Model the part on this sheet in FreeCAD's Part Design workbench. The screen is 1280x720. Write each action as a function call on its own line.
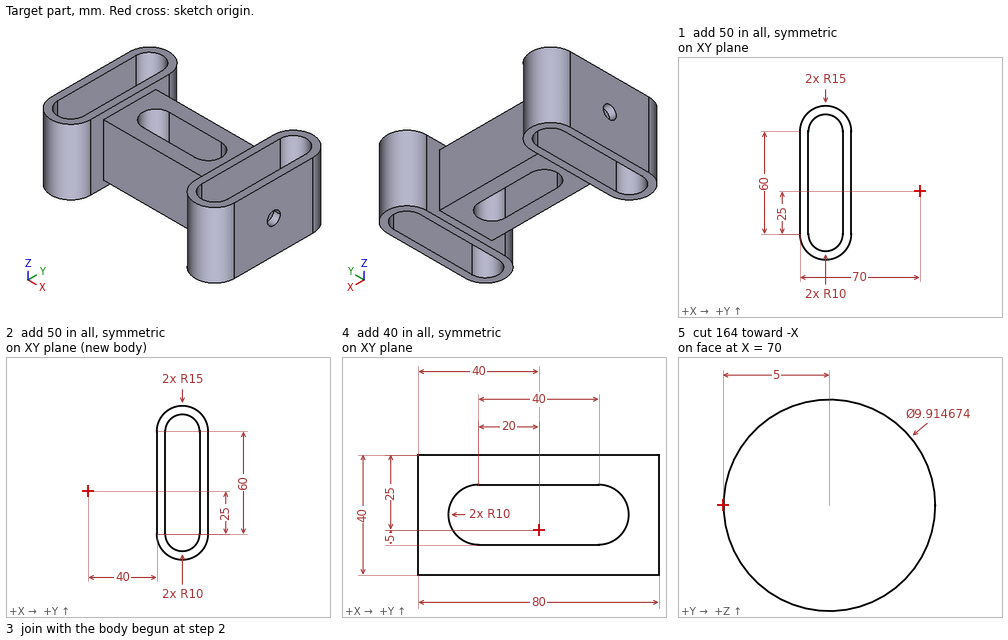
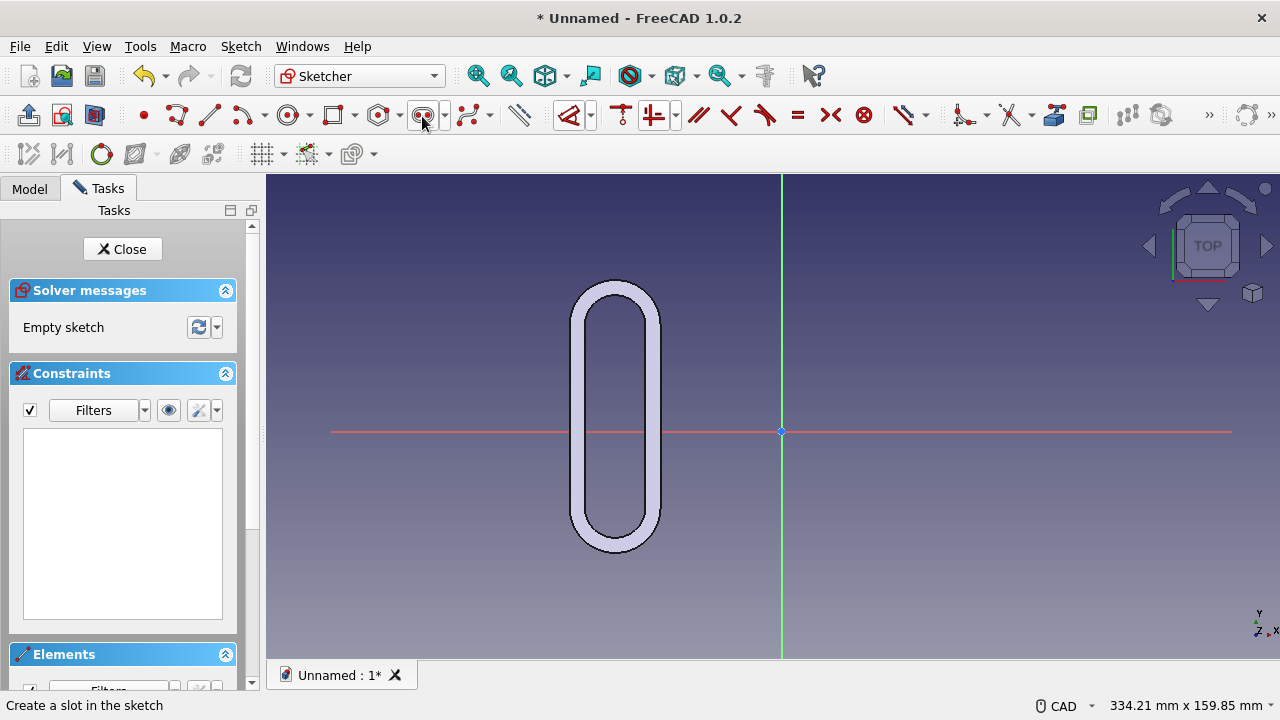
click(949, 508)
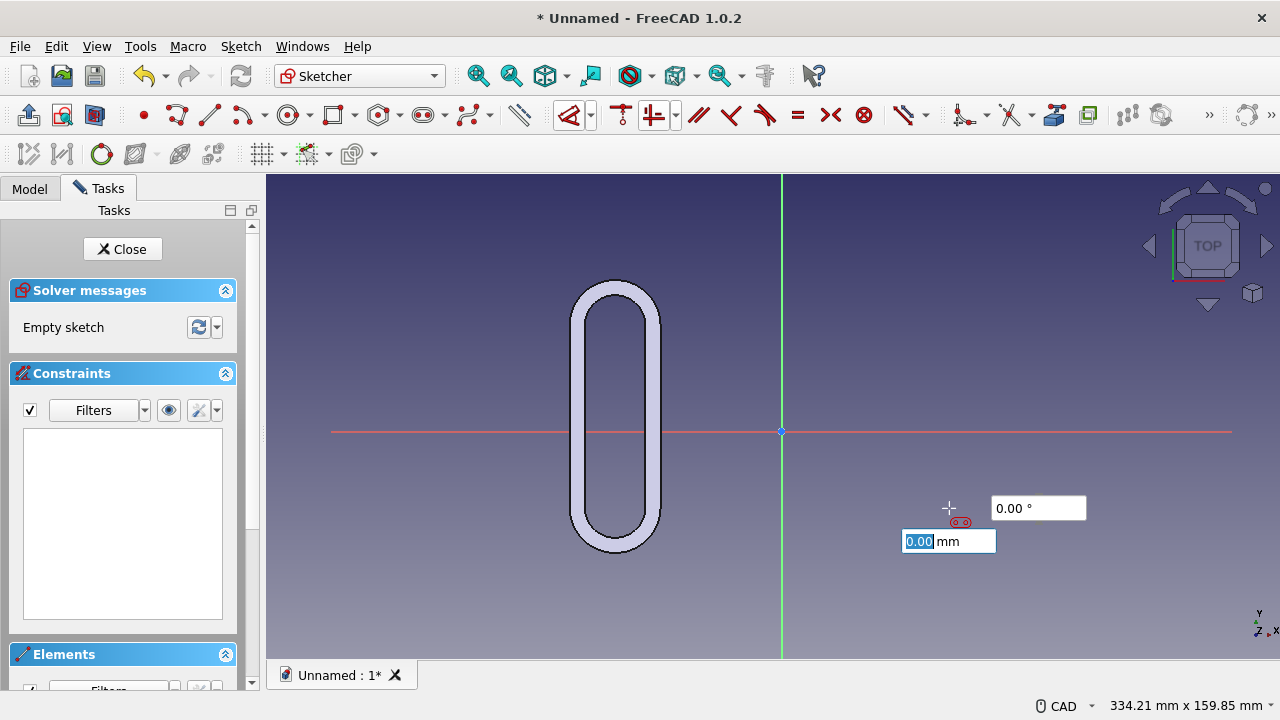
click(949, 325)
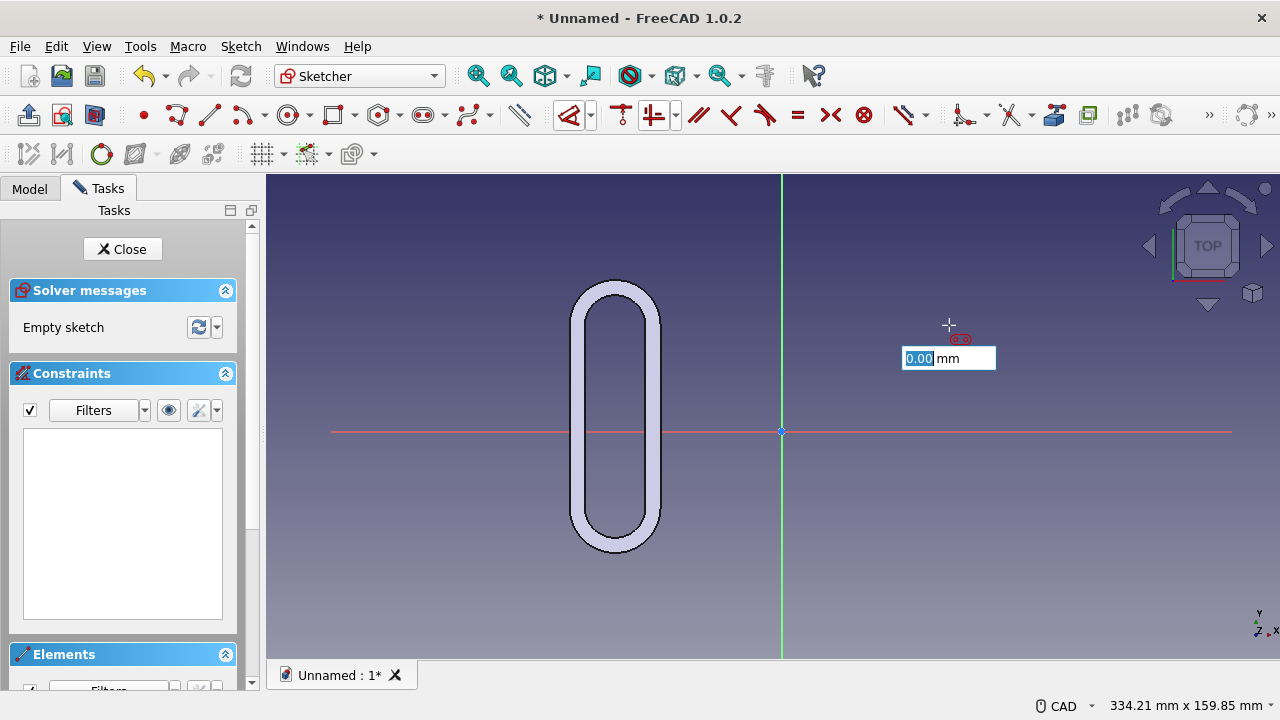
click(994, 416)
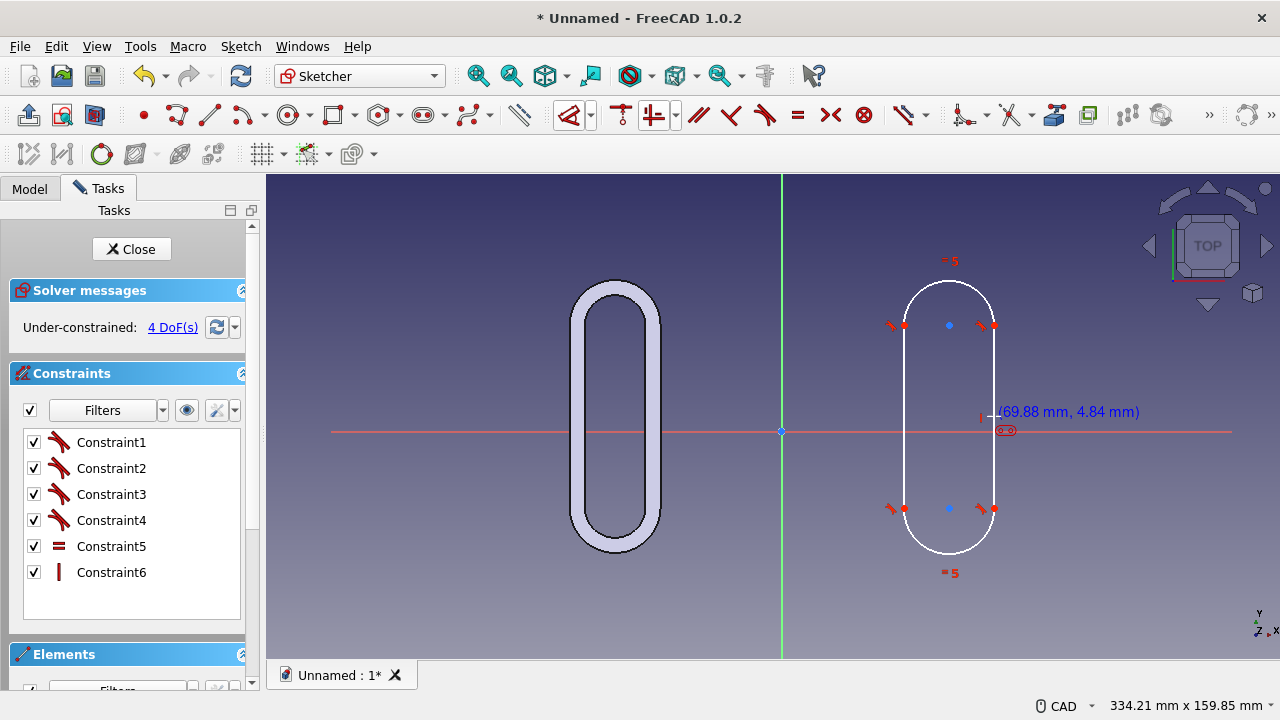
click(949, 509)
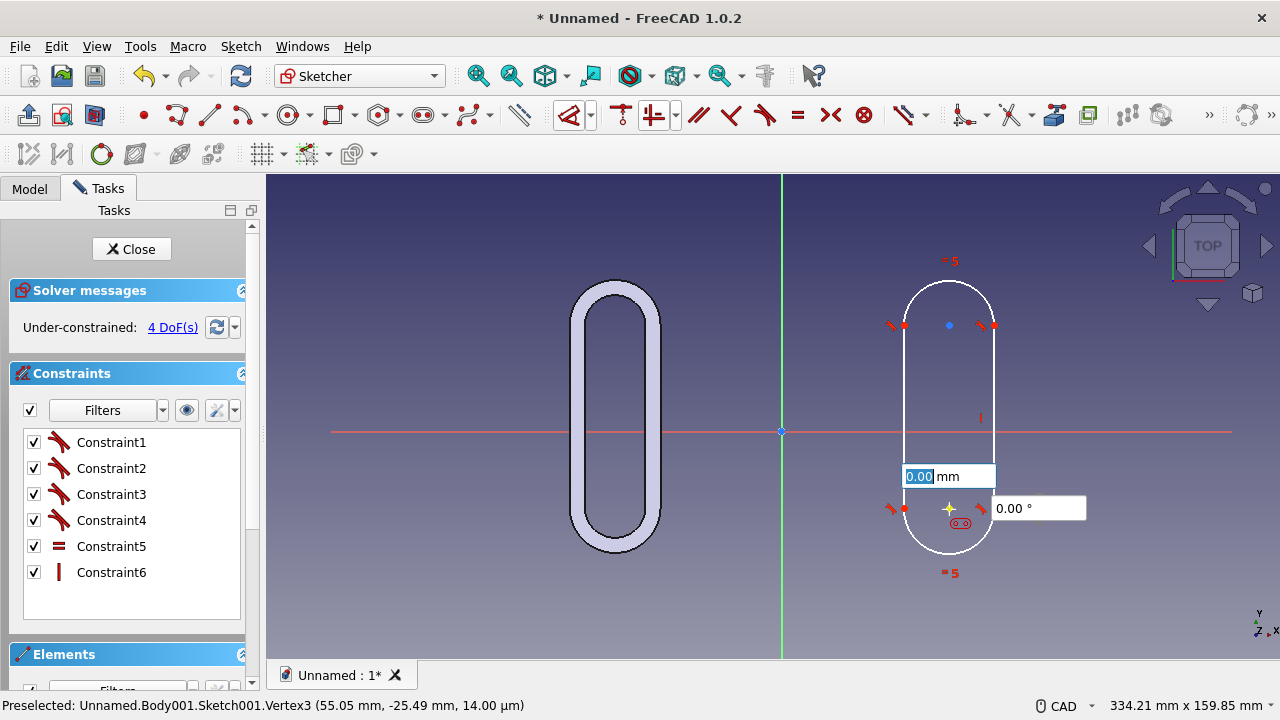
click(949, 326)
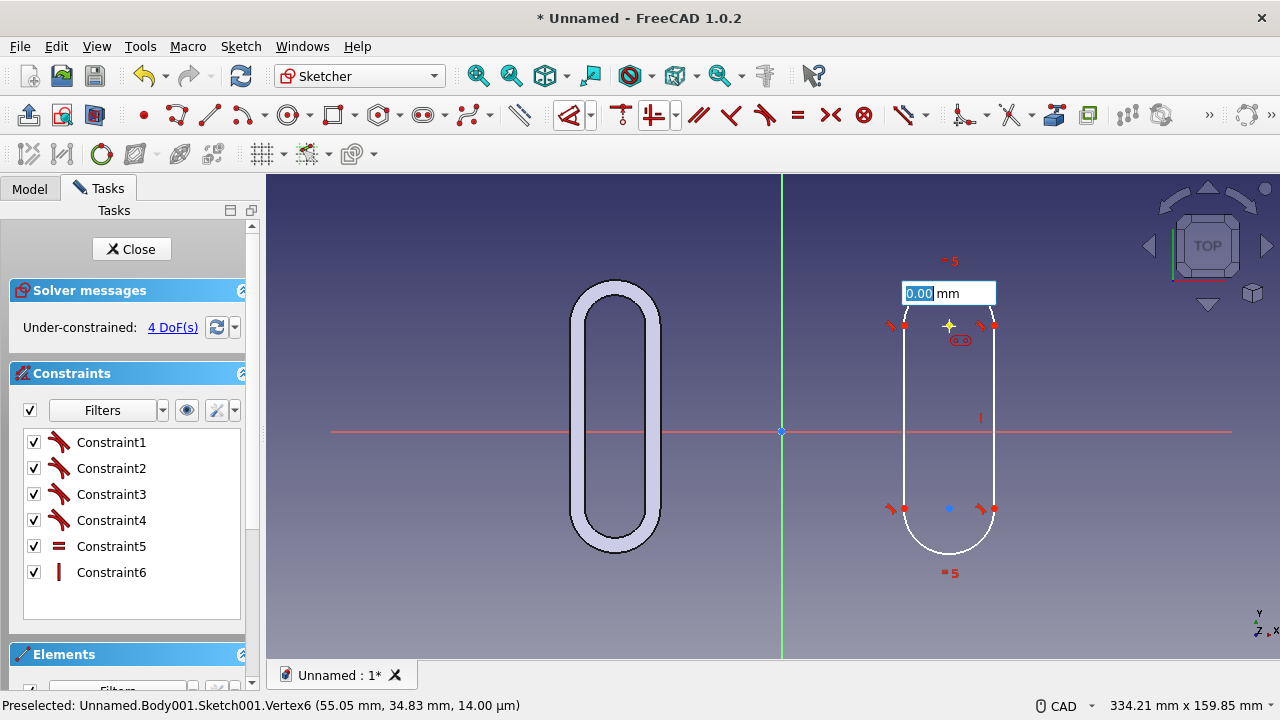
click(979, 416)
key(Escape)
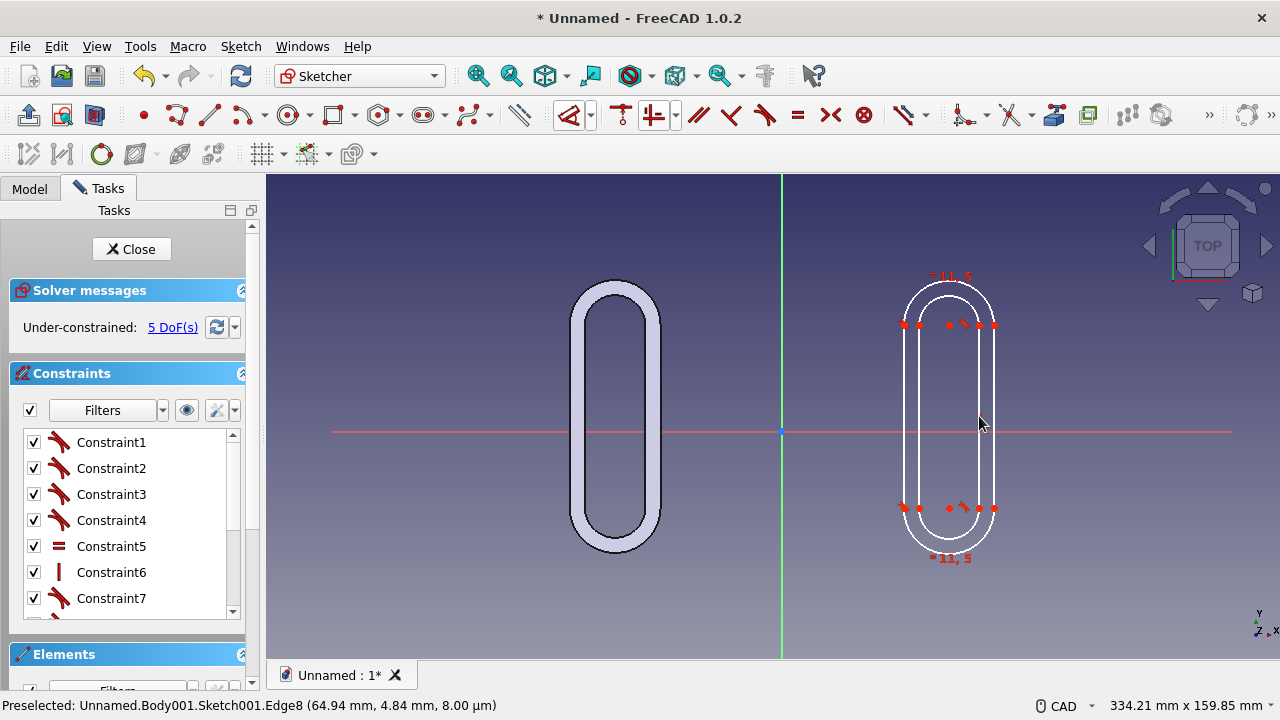
click(923, 545)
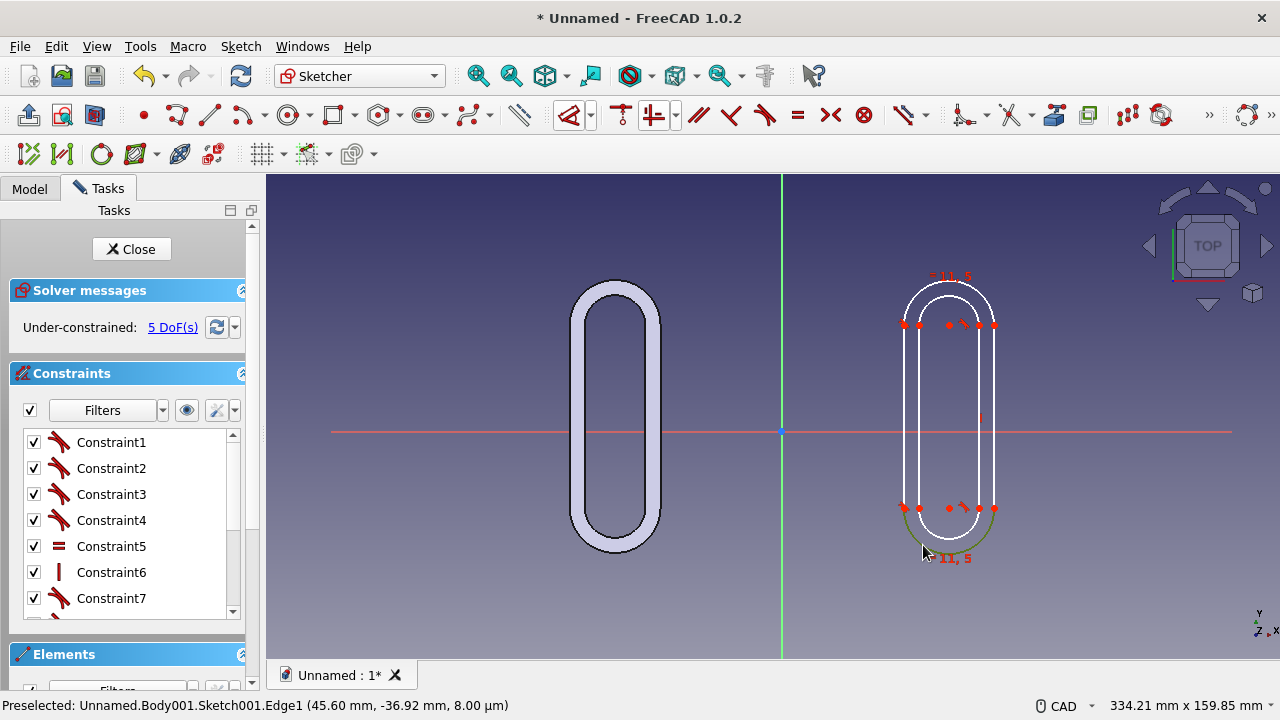
click(590, 116)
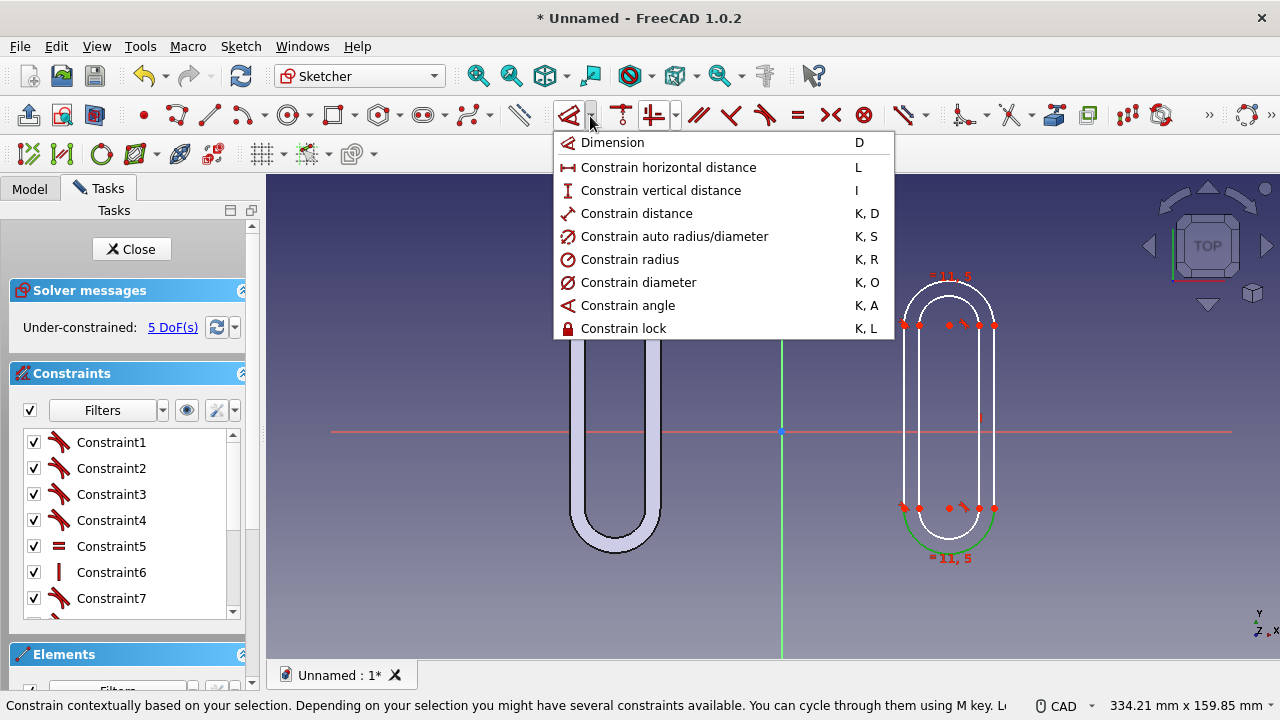
click(724, 260)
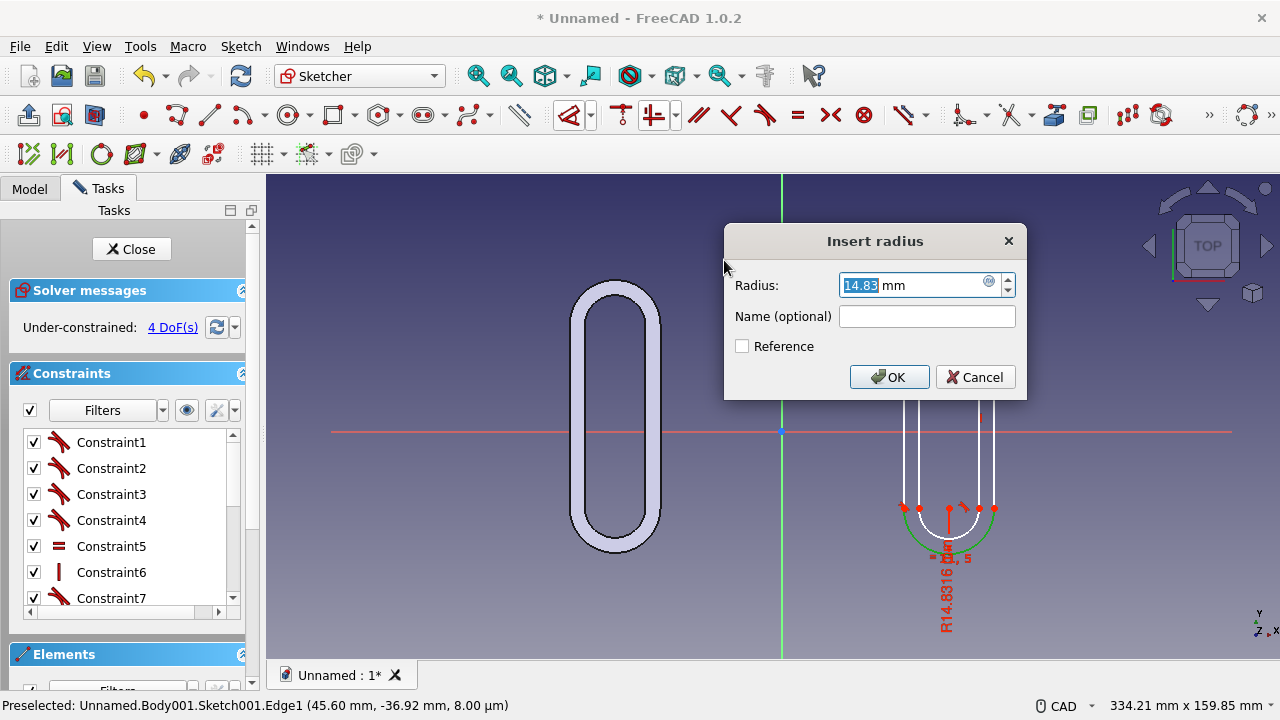
text(15)
key(Return)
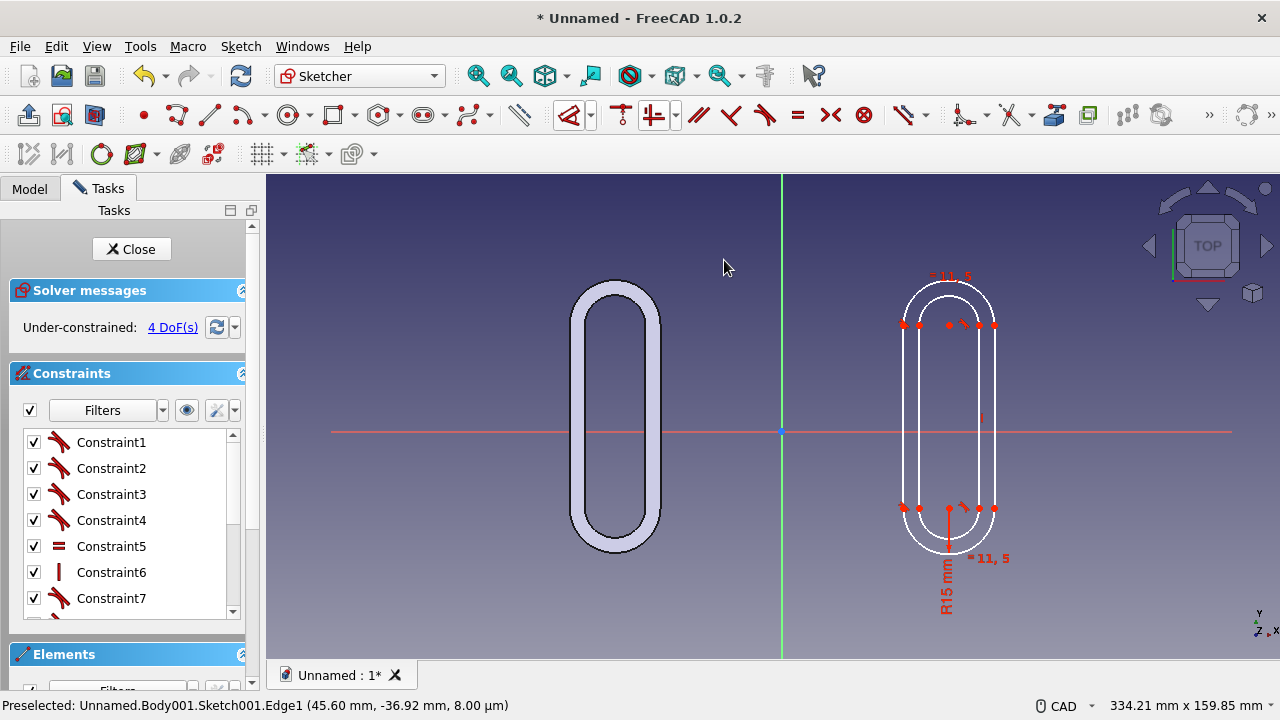
scroll(931, 533, up, 2)